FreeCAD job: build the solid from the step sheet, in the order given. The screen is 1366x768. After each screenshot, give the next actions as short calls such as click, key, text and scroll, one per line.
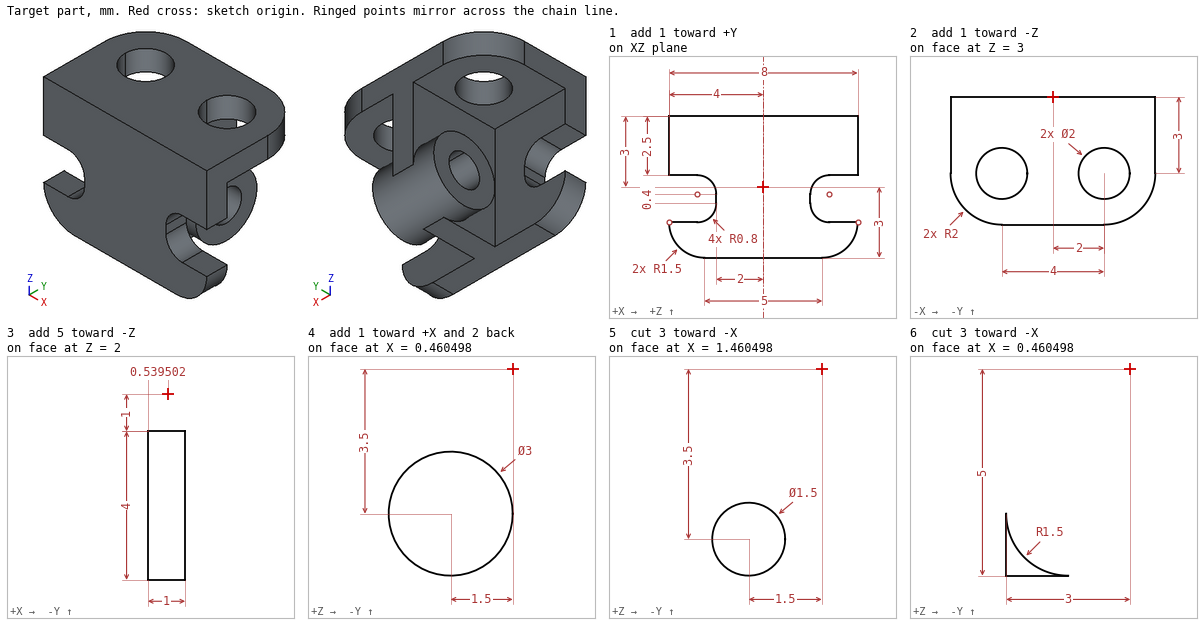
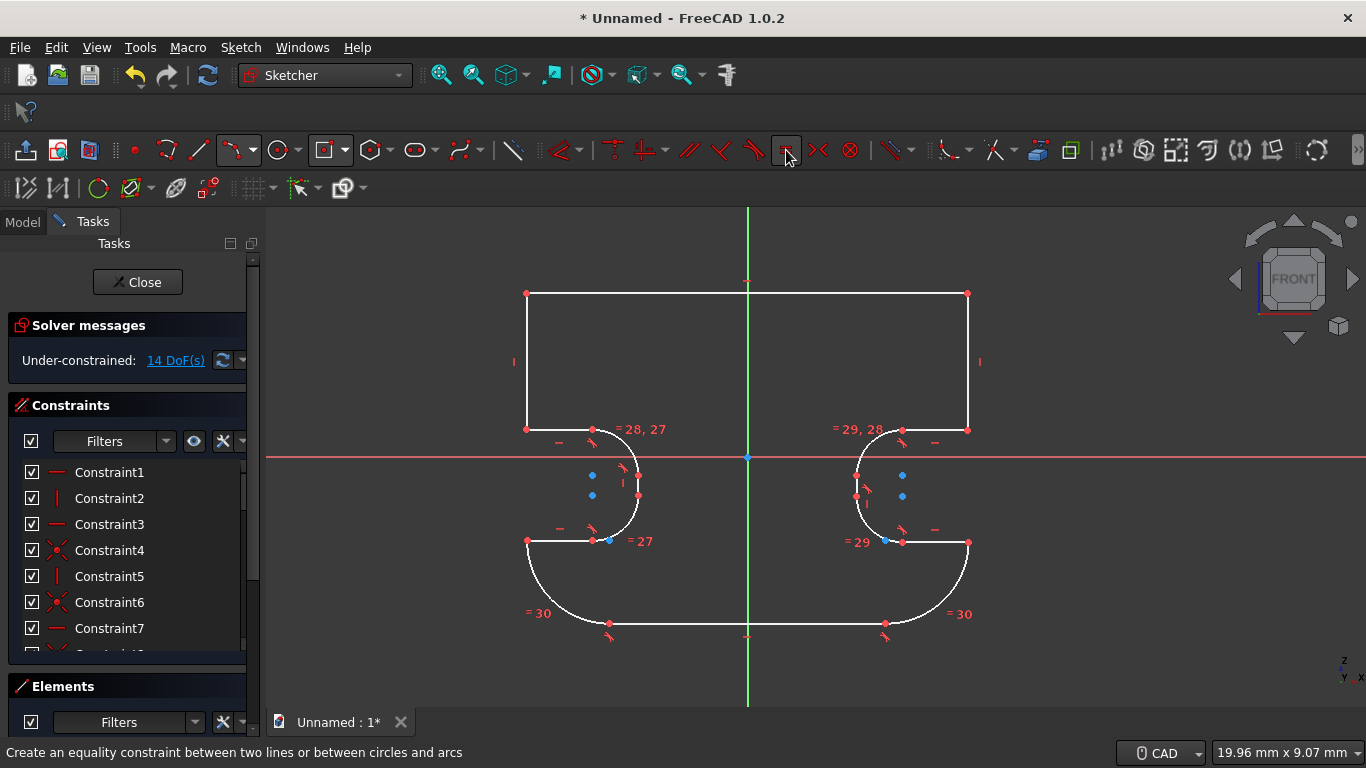
click(593, 475)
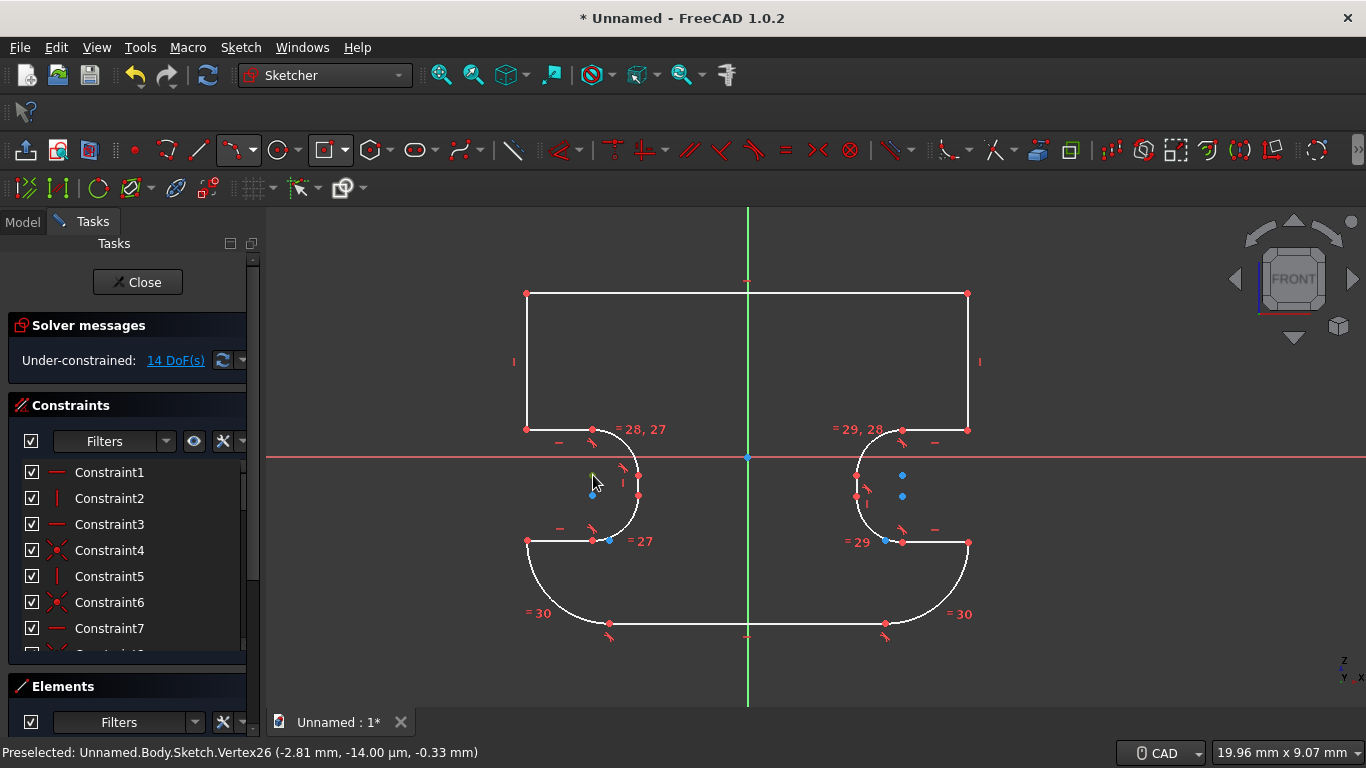
click(902, 476)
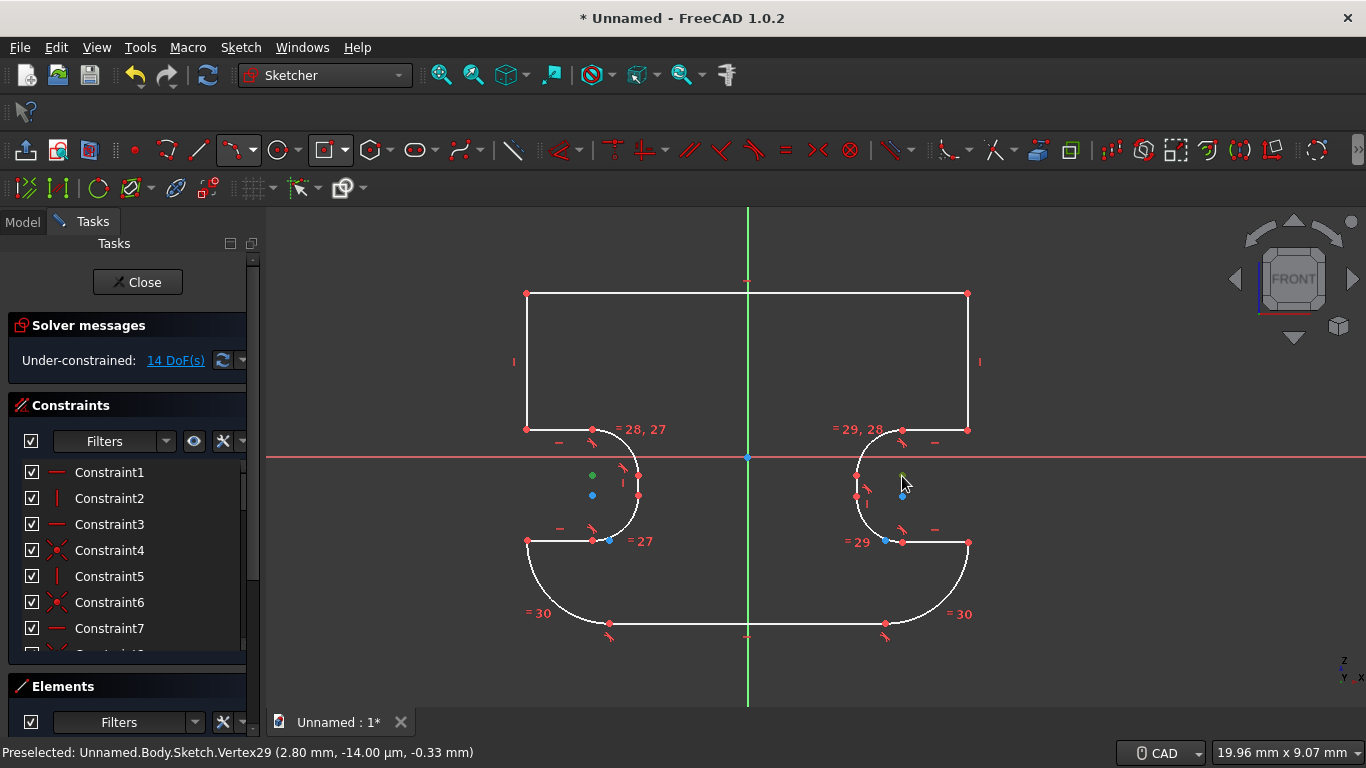
click(748, 584)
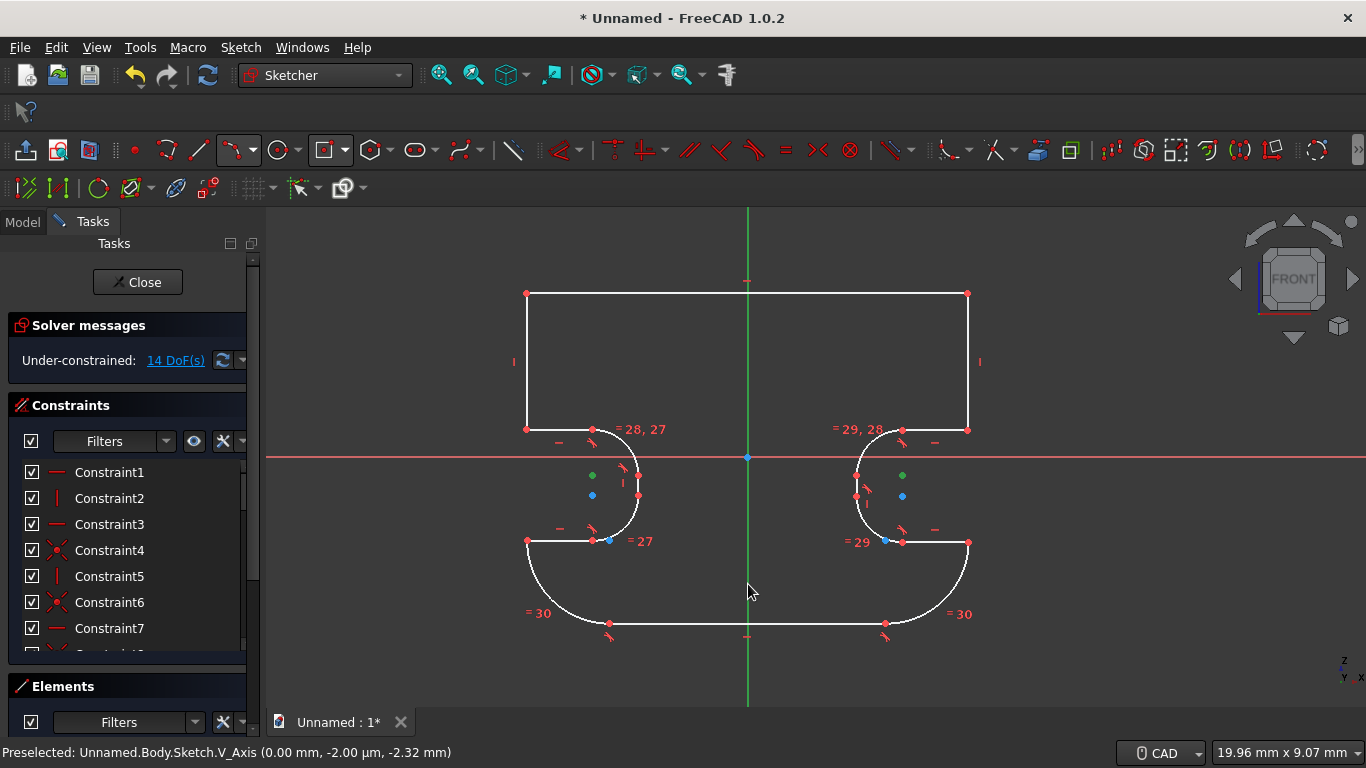
click(818, 150)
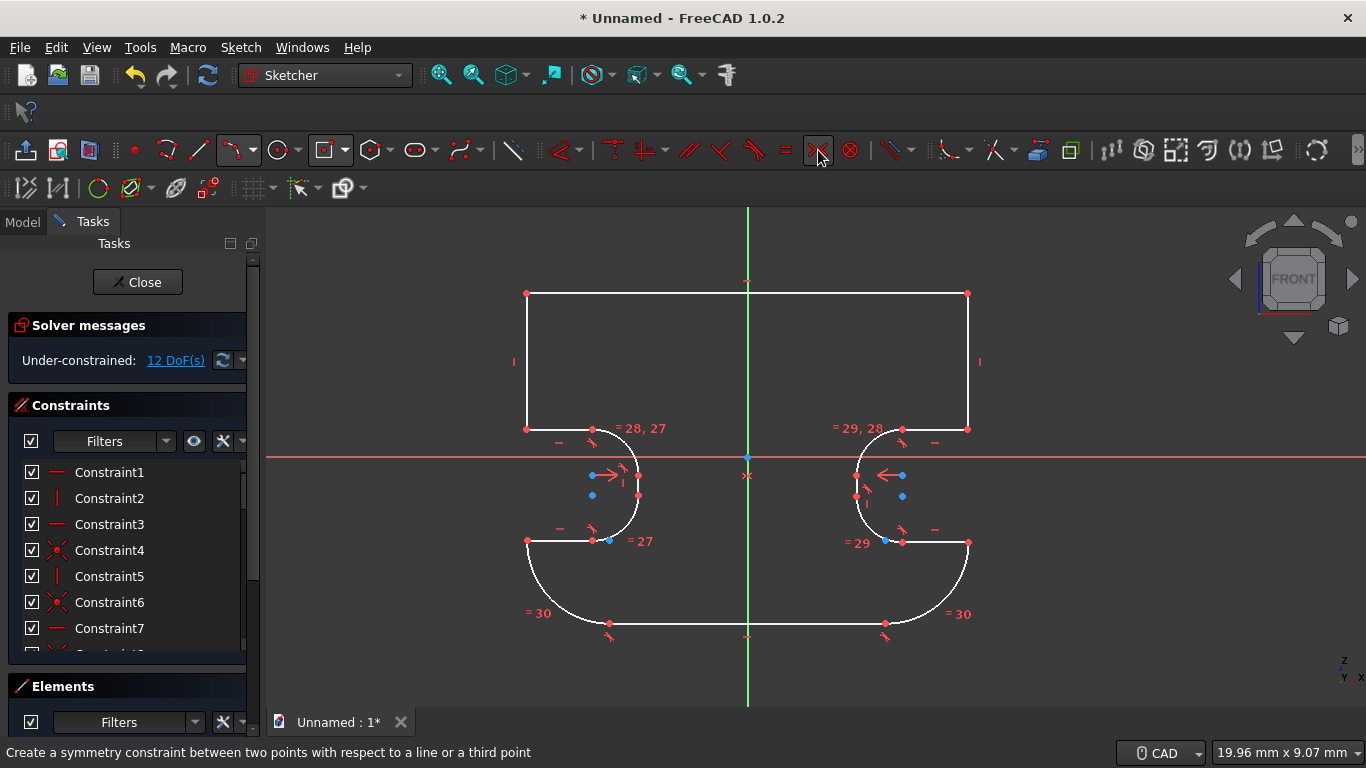
click(527, 541)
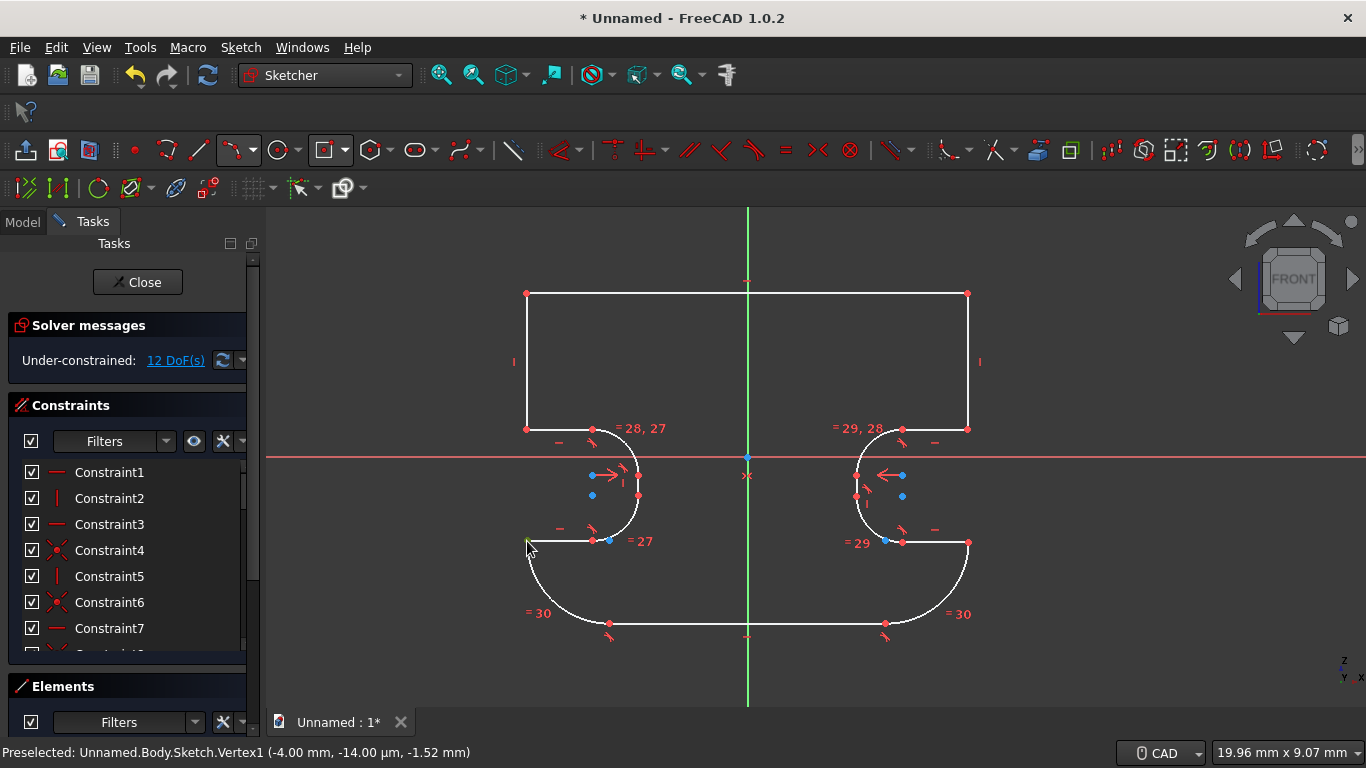
click(969, 542)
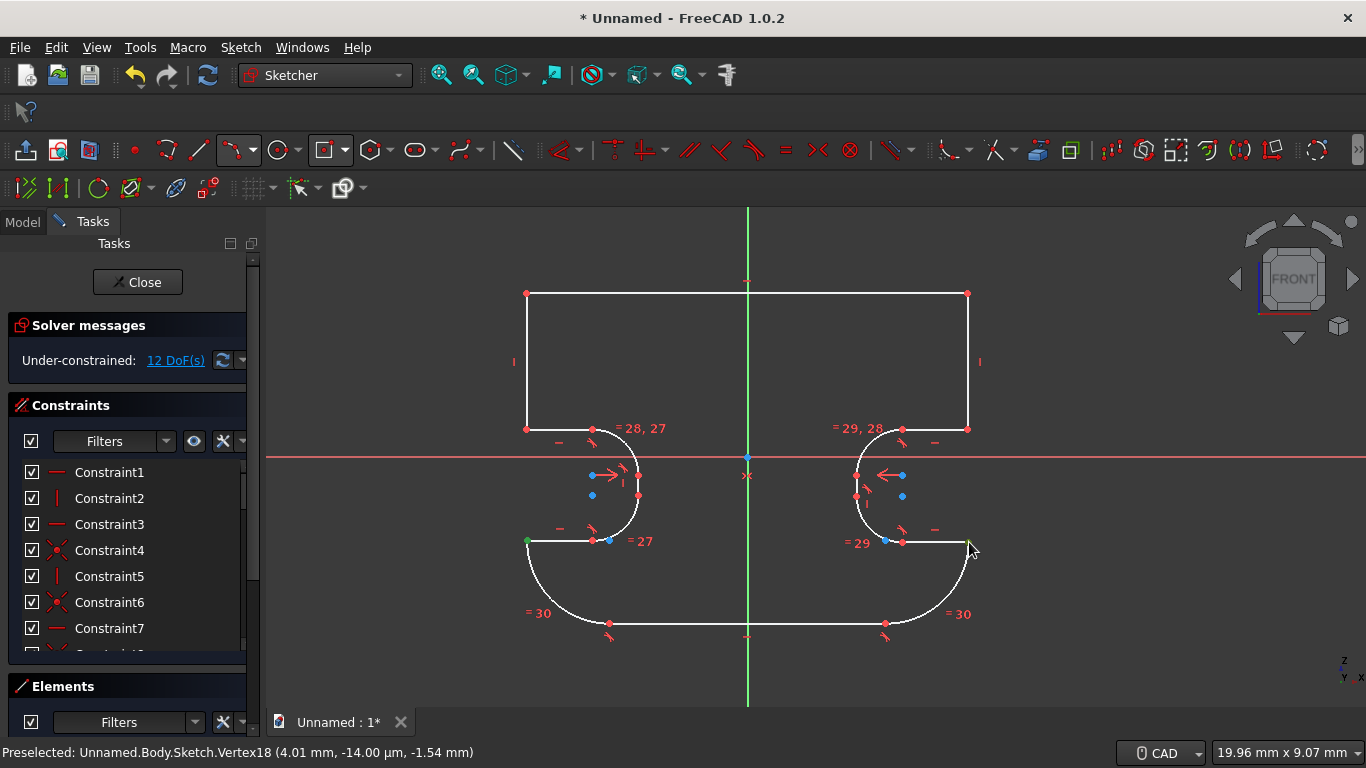
click(748, 584)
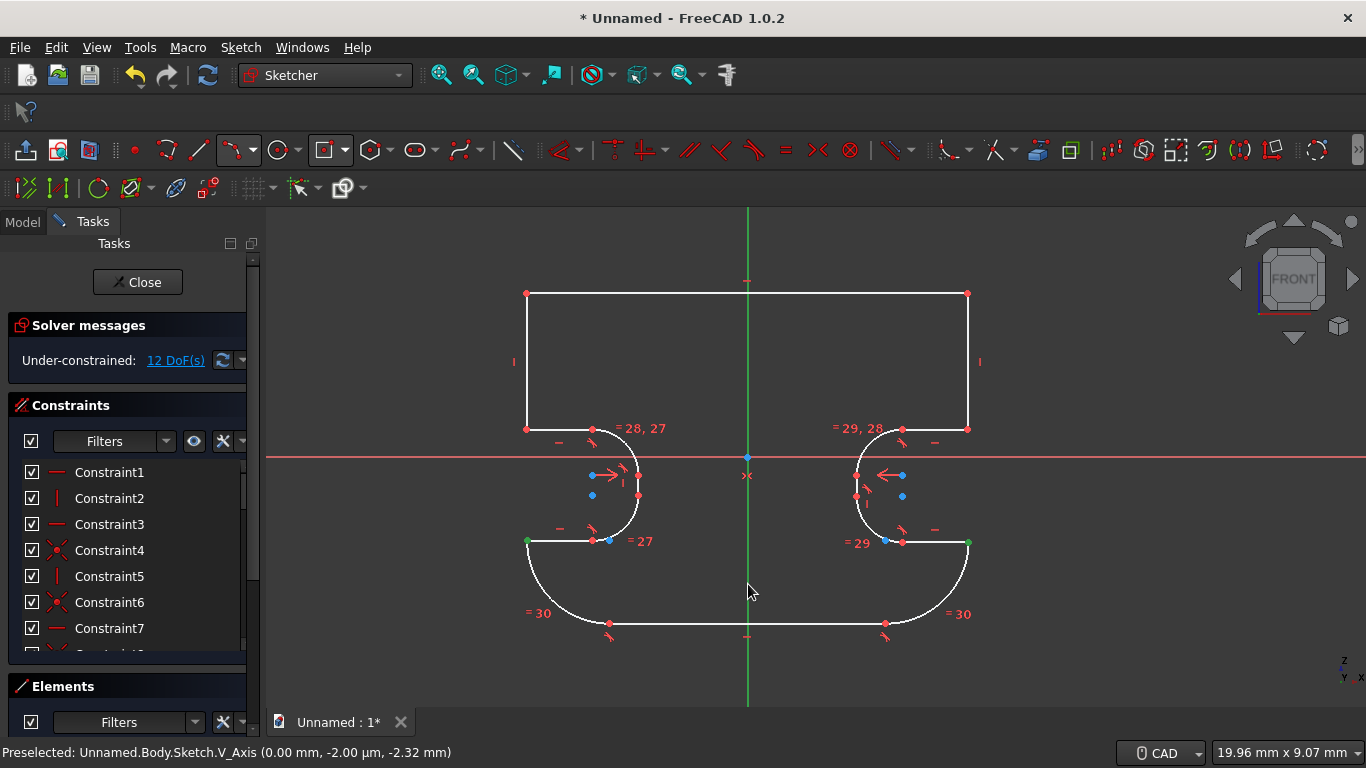
click(818, 150)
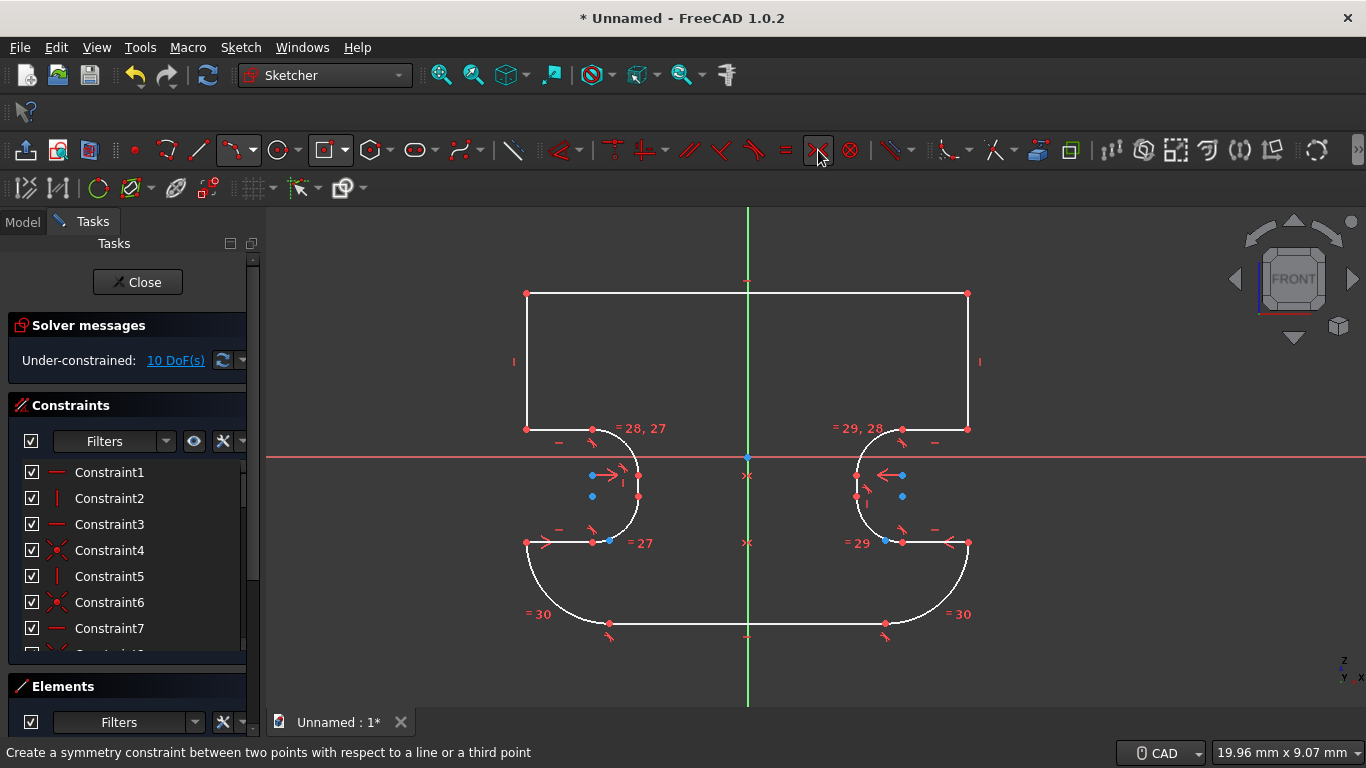
click(560, 150)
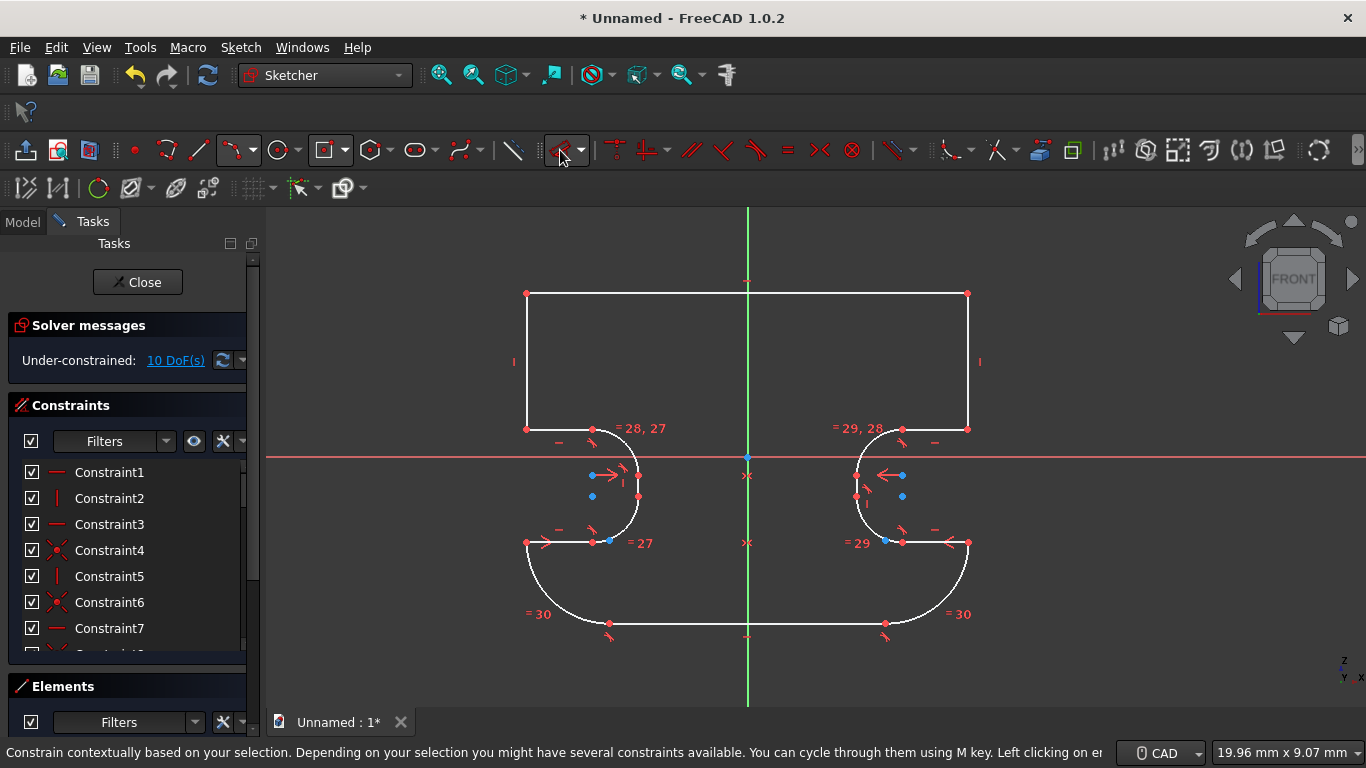
click(614, 537)
click(629, 565)